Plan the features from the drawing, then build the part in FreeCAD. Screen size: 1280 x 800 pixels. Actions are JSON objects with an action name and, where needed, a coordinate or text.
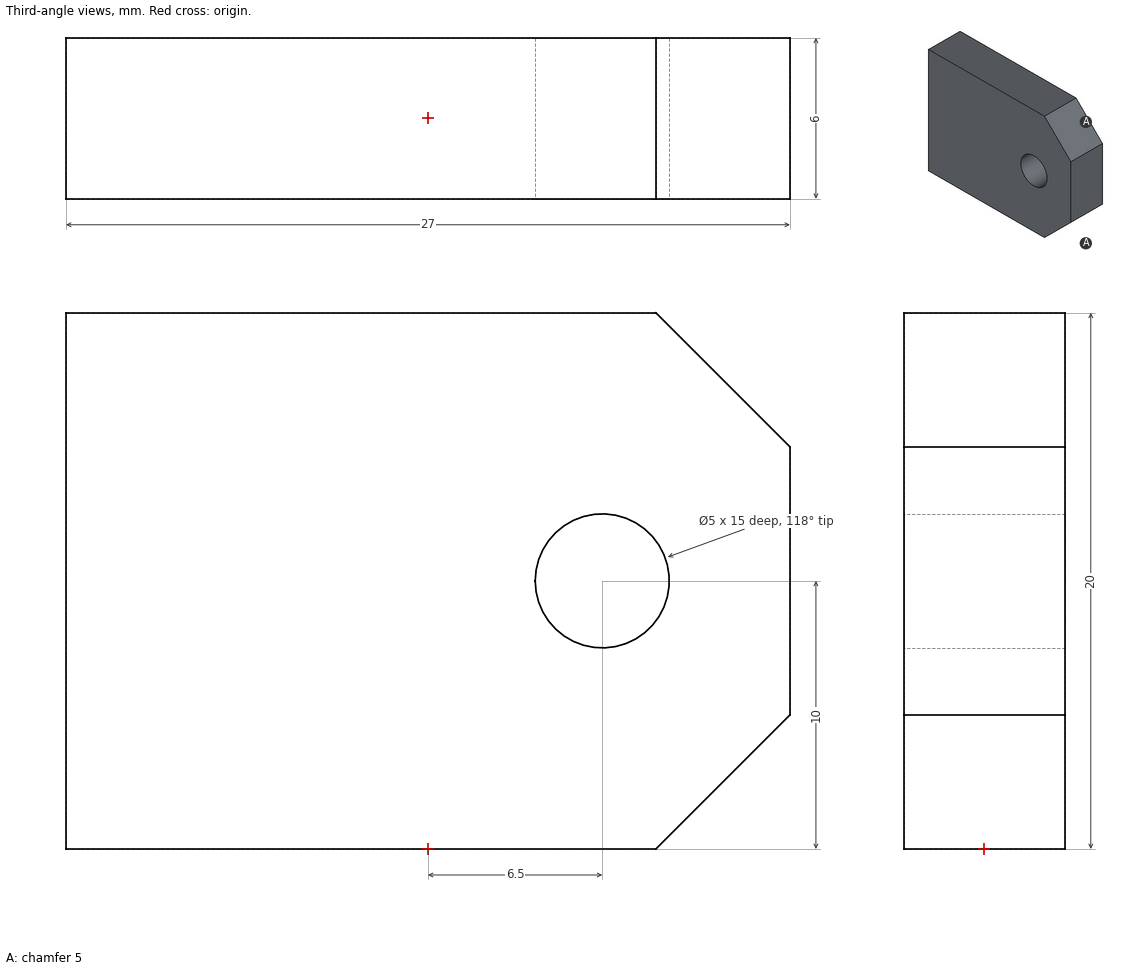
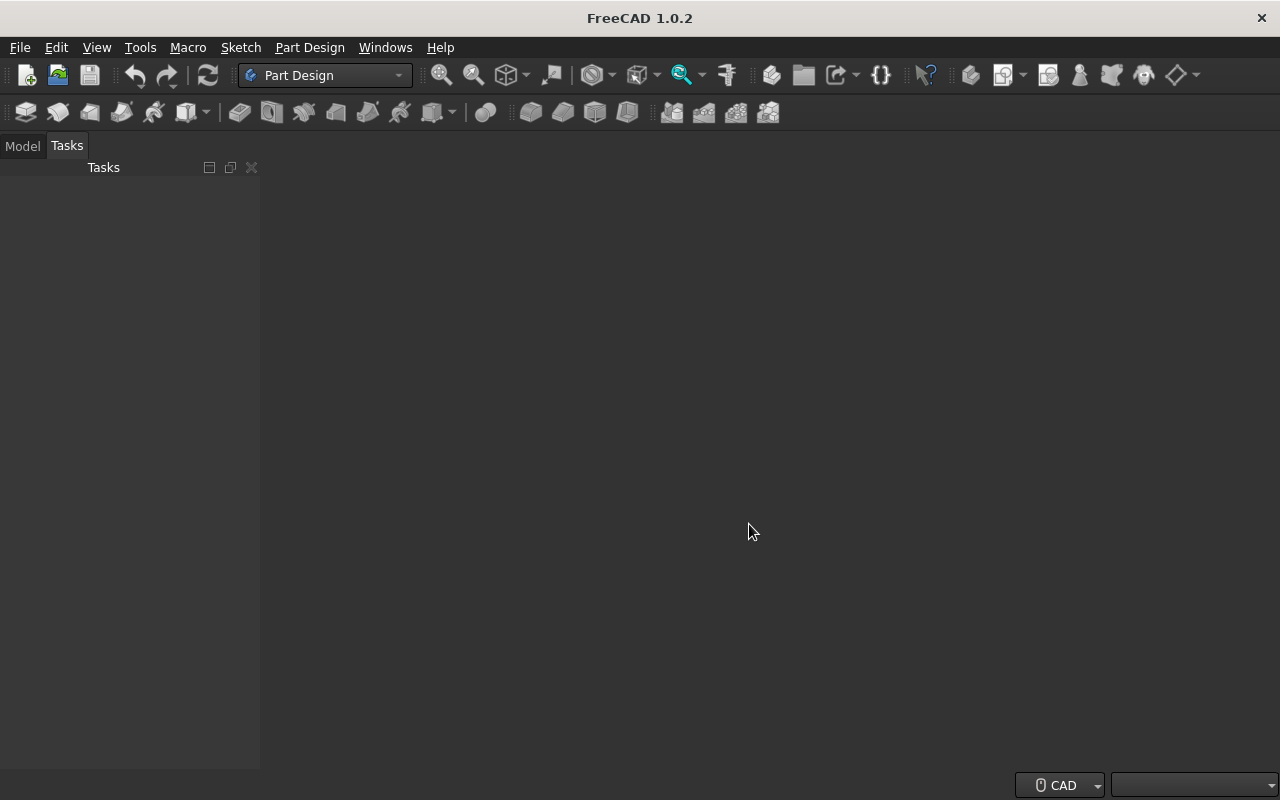
{"action": "left_click", "coordinate": [26, 76]}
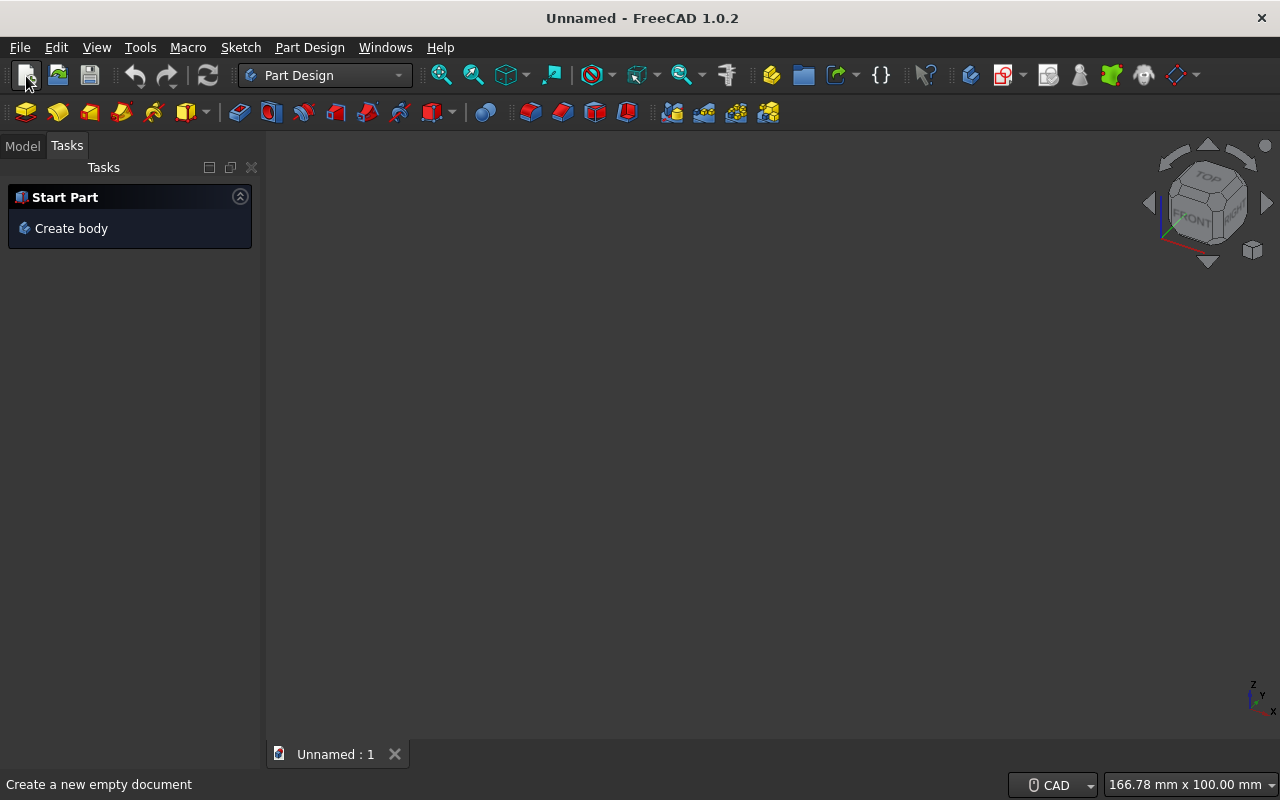
{"action": "left_click", "coordinate": [1004, 76]}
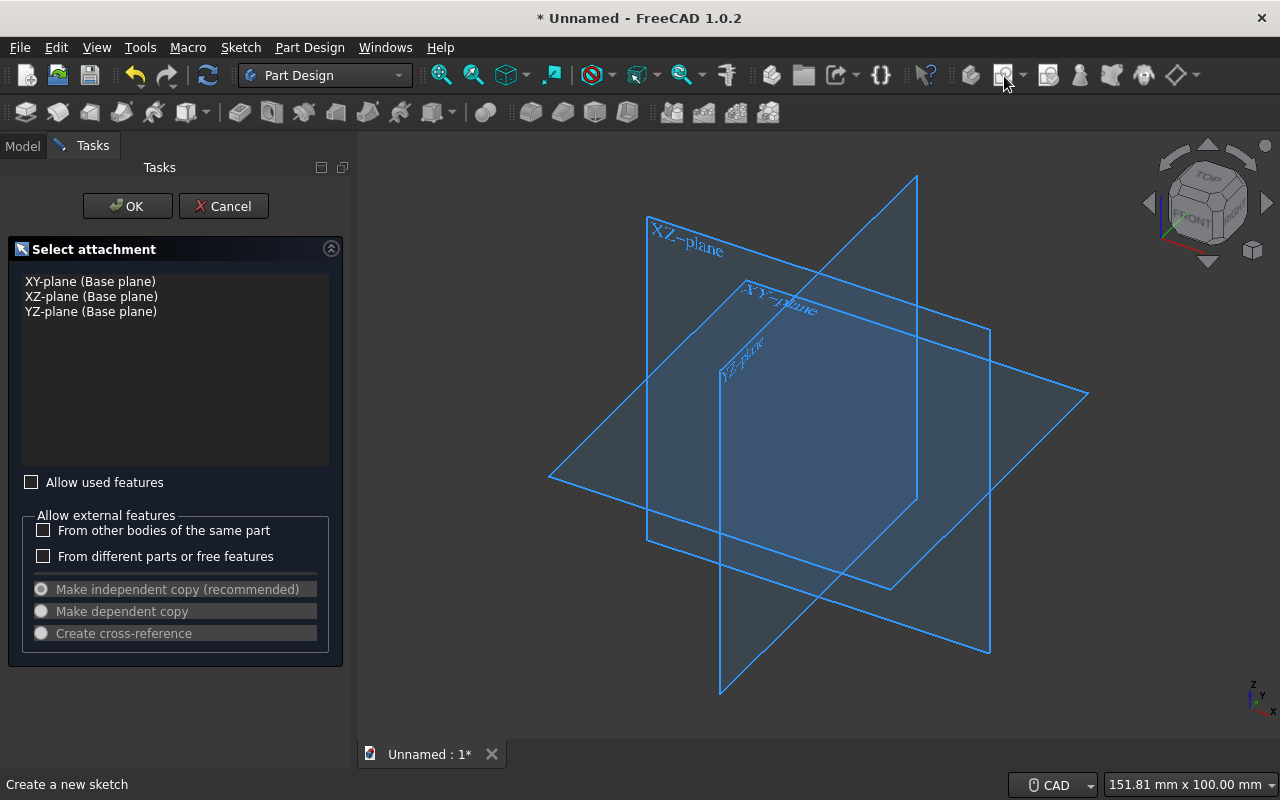
{"action": "left_click", "coordinate": [82, 282]}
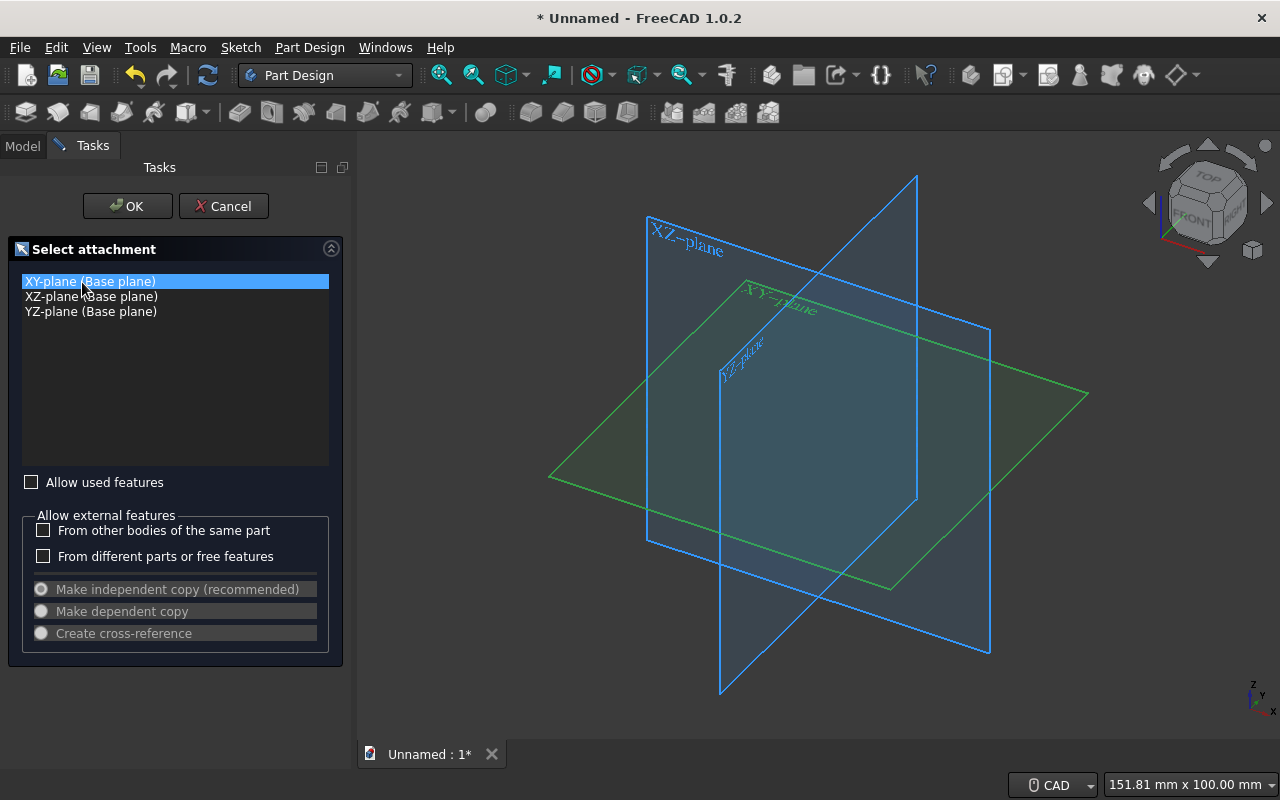
{"action": "left_click", "coordinate": [128, 206]}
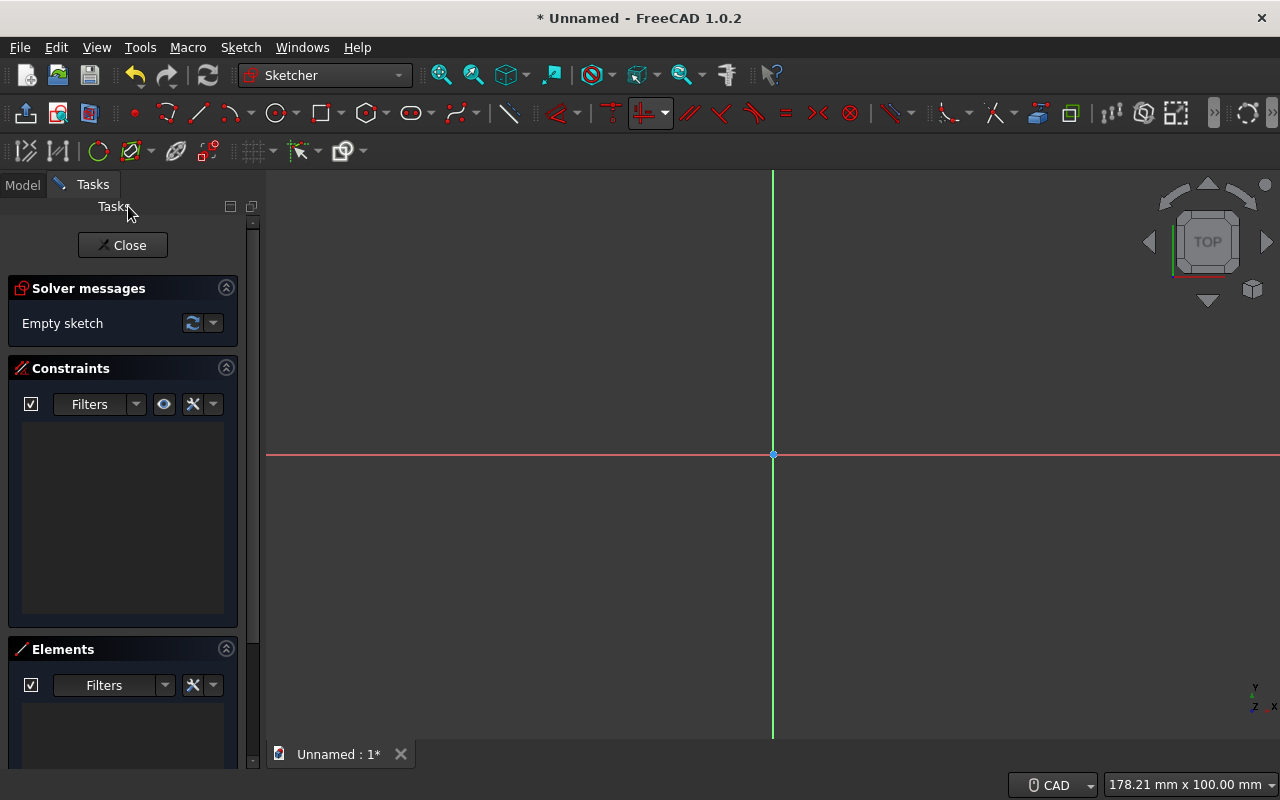
{"action": "scroll", "coordinate": [795, 454], "scroll_direction": "up", "scroll_amount": 7}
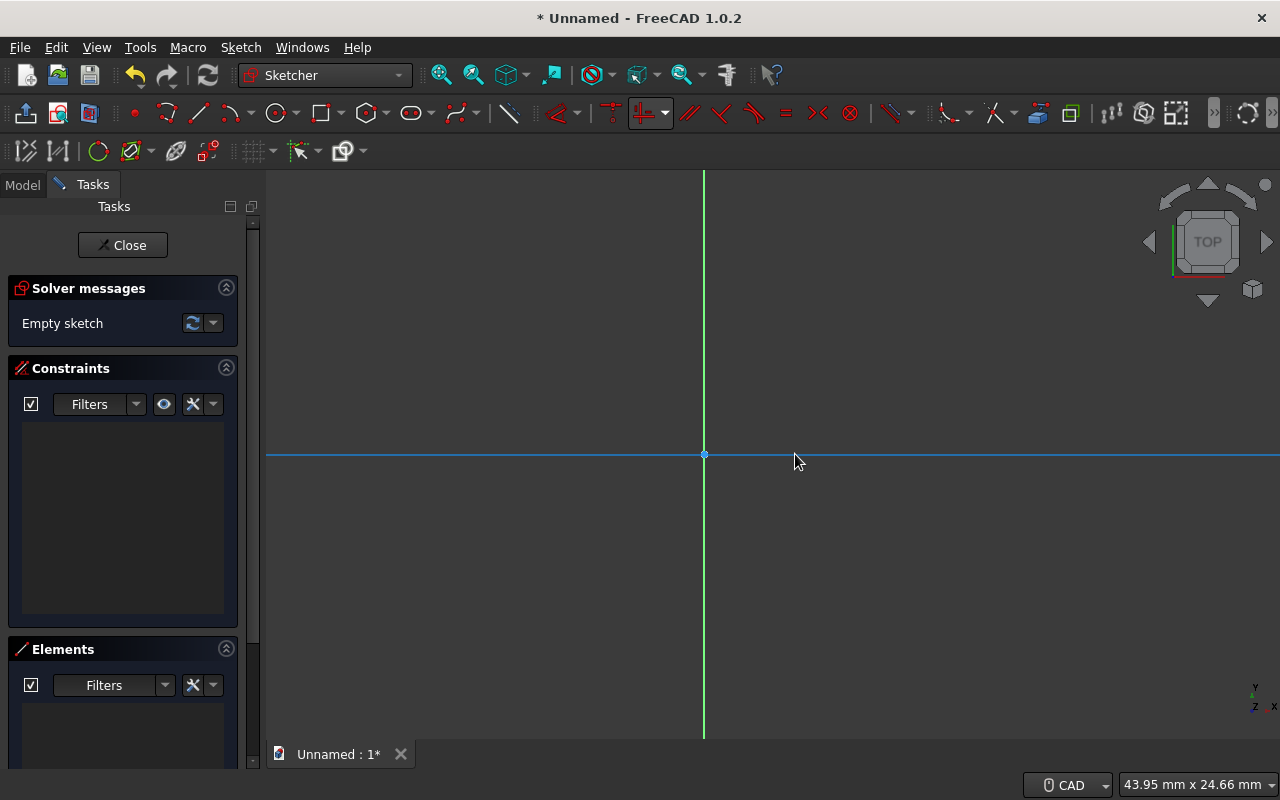
{"action": "left_click", "coordinate": [344, 114]}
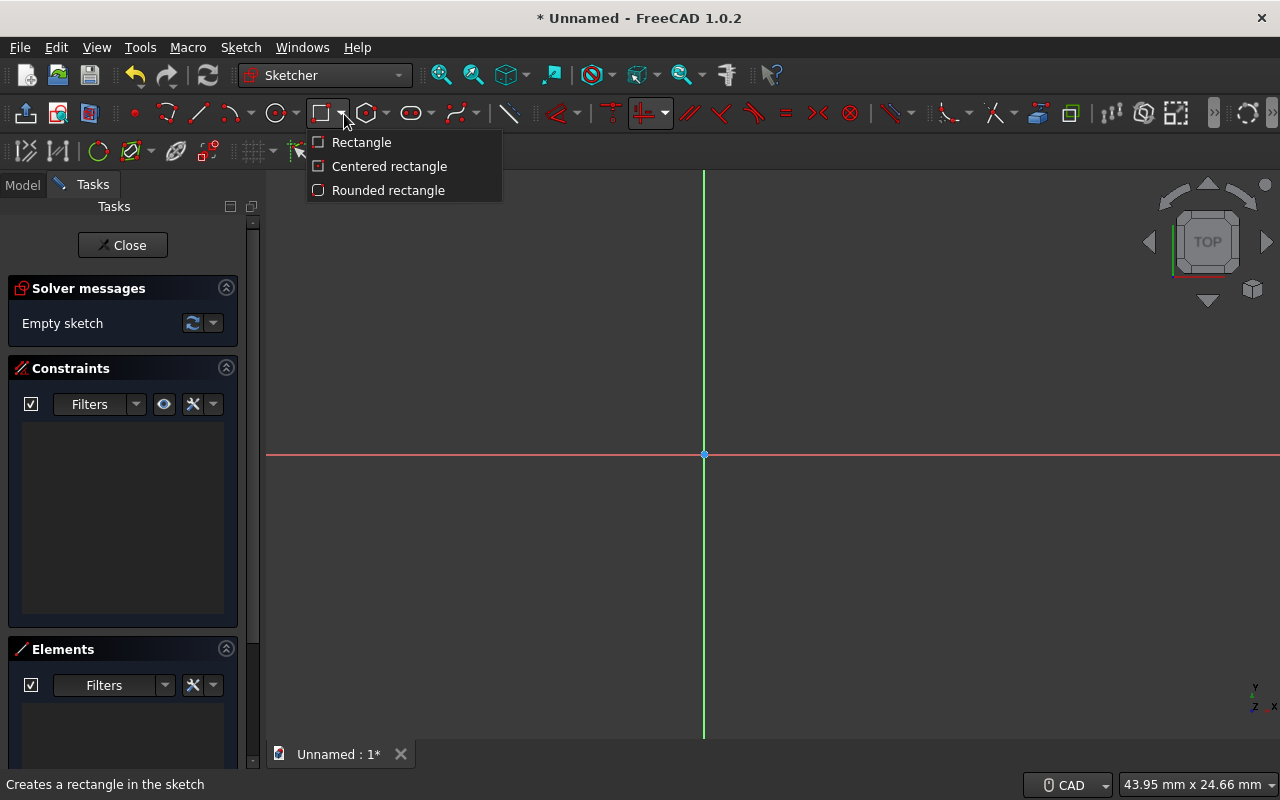
{"action": "left_click", "coordinate": [404, 166]}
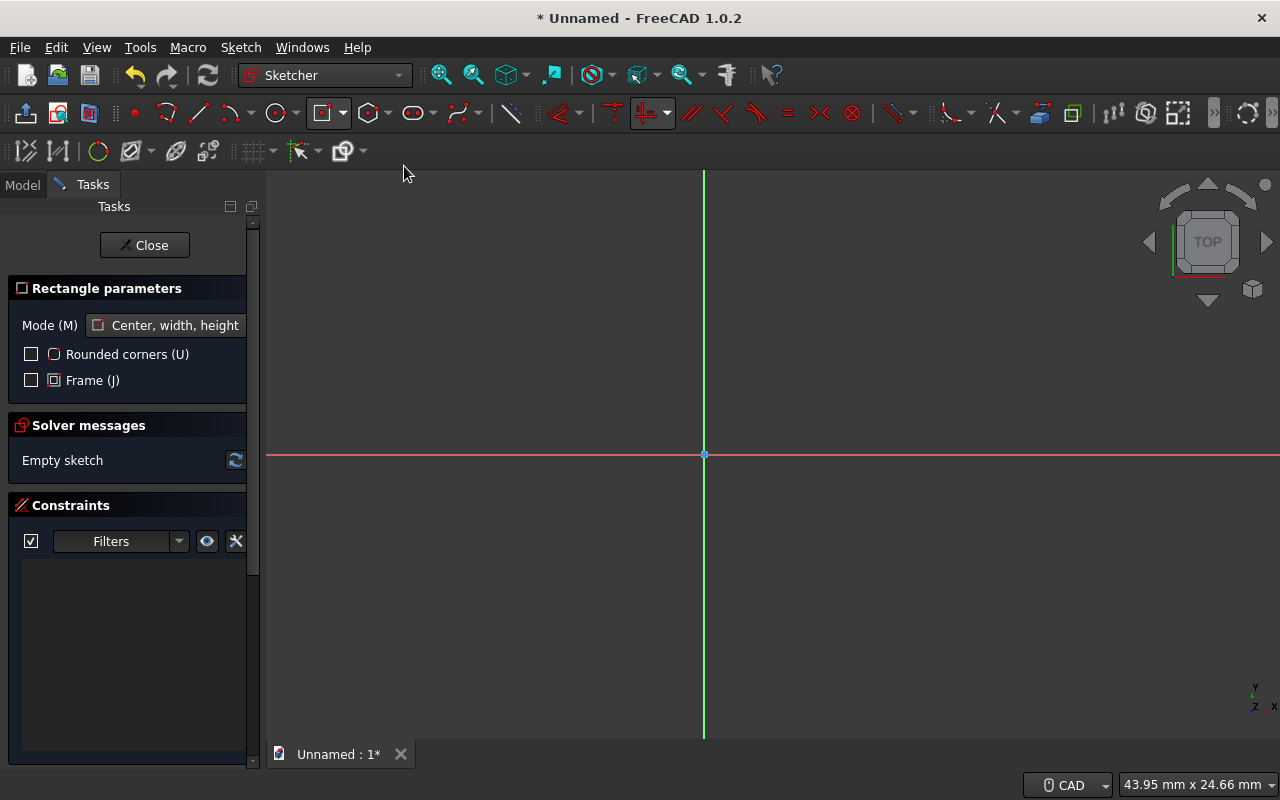
{"action": "left_click", "coordinate": [704, 454]}
{"action": "left_click", "coordinate": [1016, 385]}
{"action": "key", "text": "Escape"}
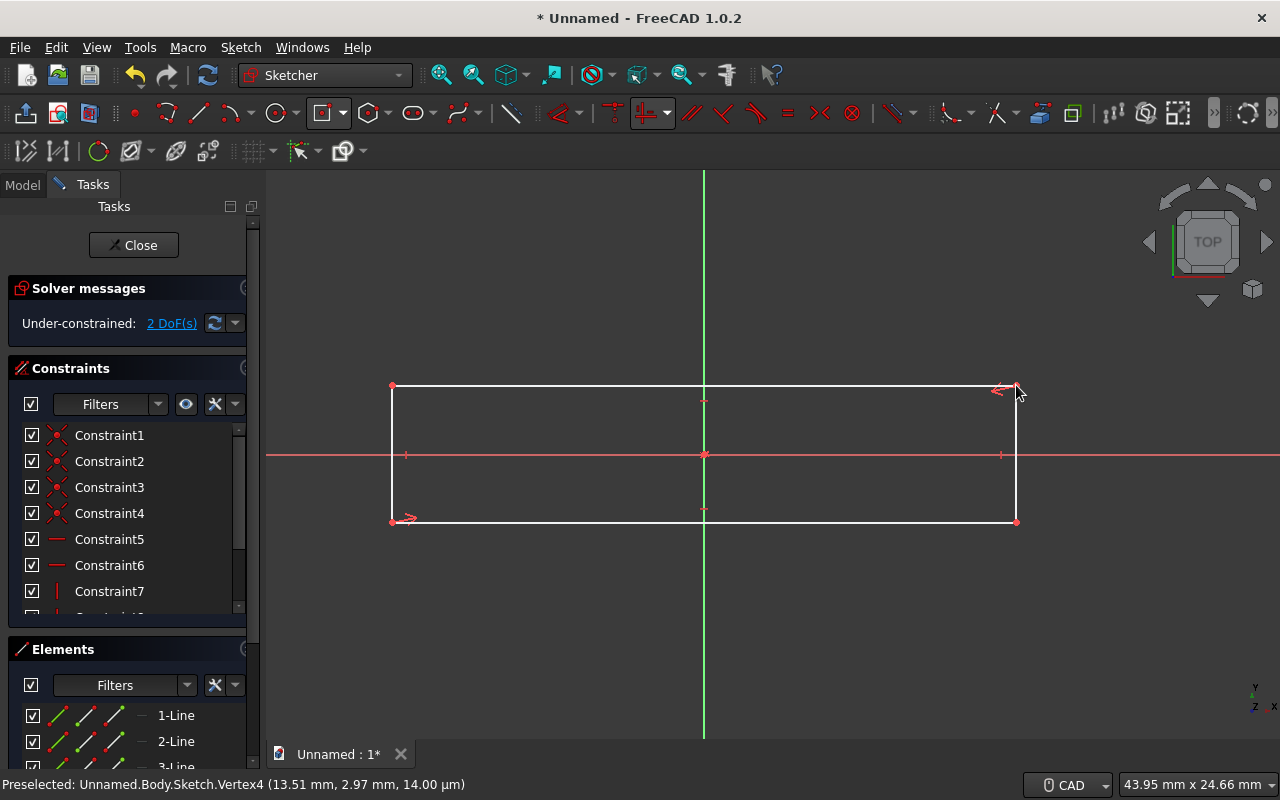
{"action": "left_click", "coordinate": [558, 114]}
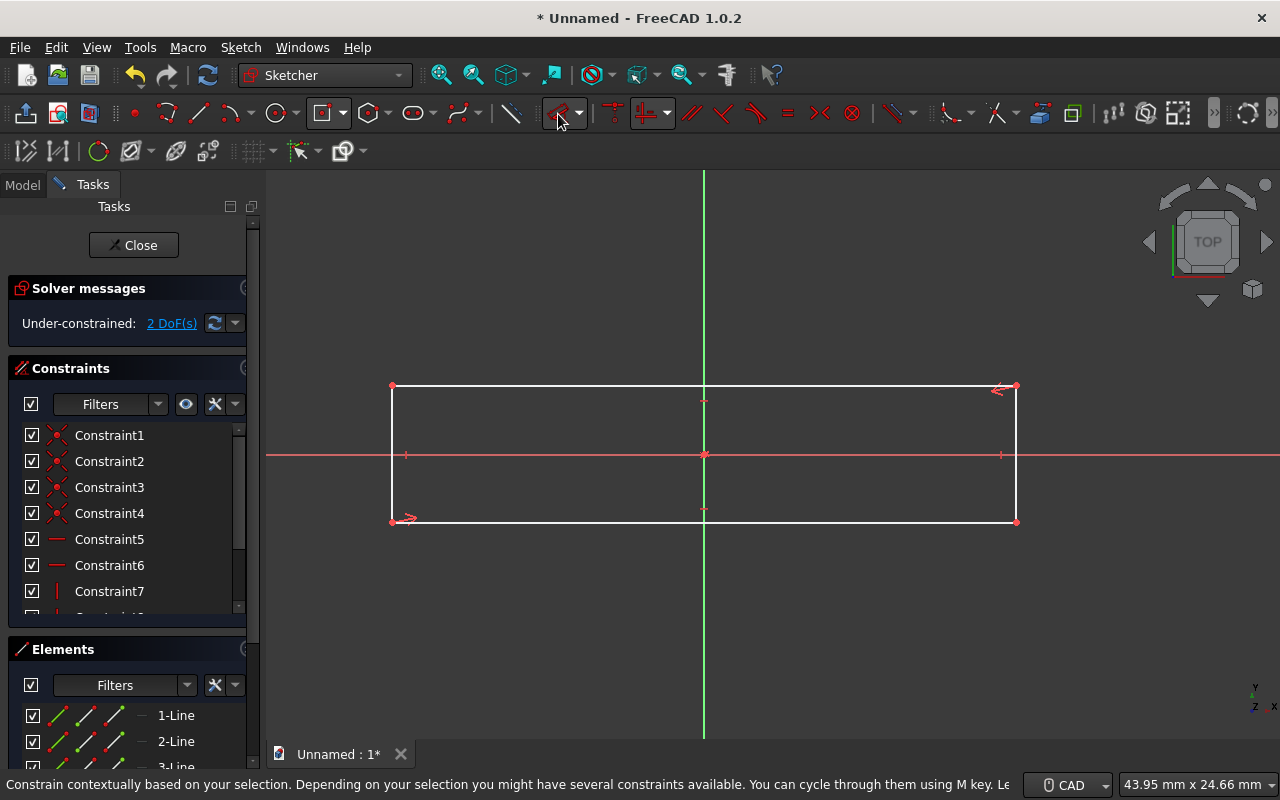
{"action": "left_click", "coordinate": [1016, 482]}
{"action": "left_click", "coordinate": [1050, 423]}